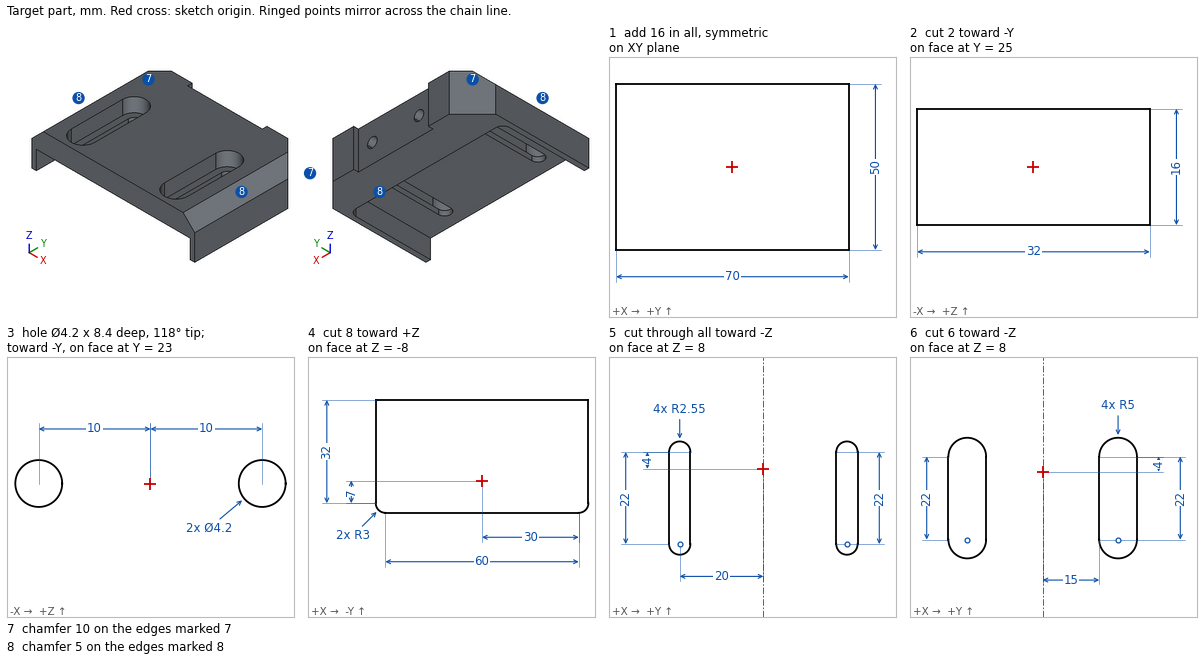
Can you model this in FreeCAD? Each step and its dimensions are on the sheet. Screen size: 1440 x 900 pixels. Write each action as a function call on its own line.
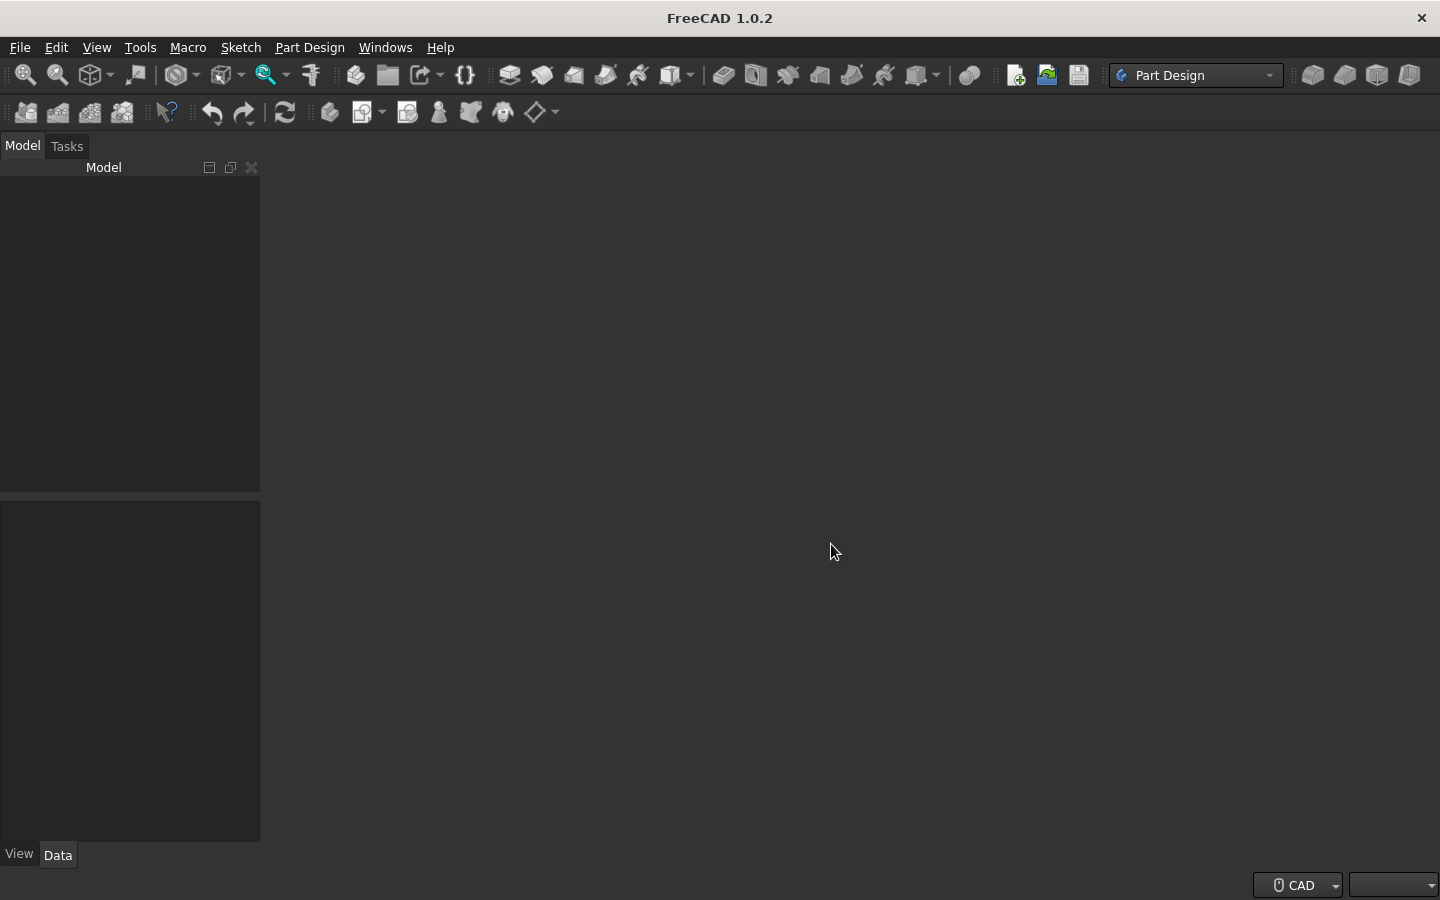
key(ctrl+n)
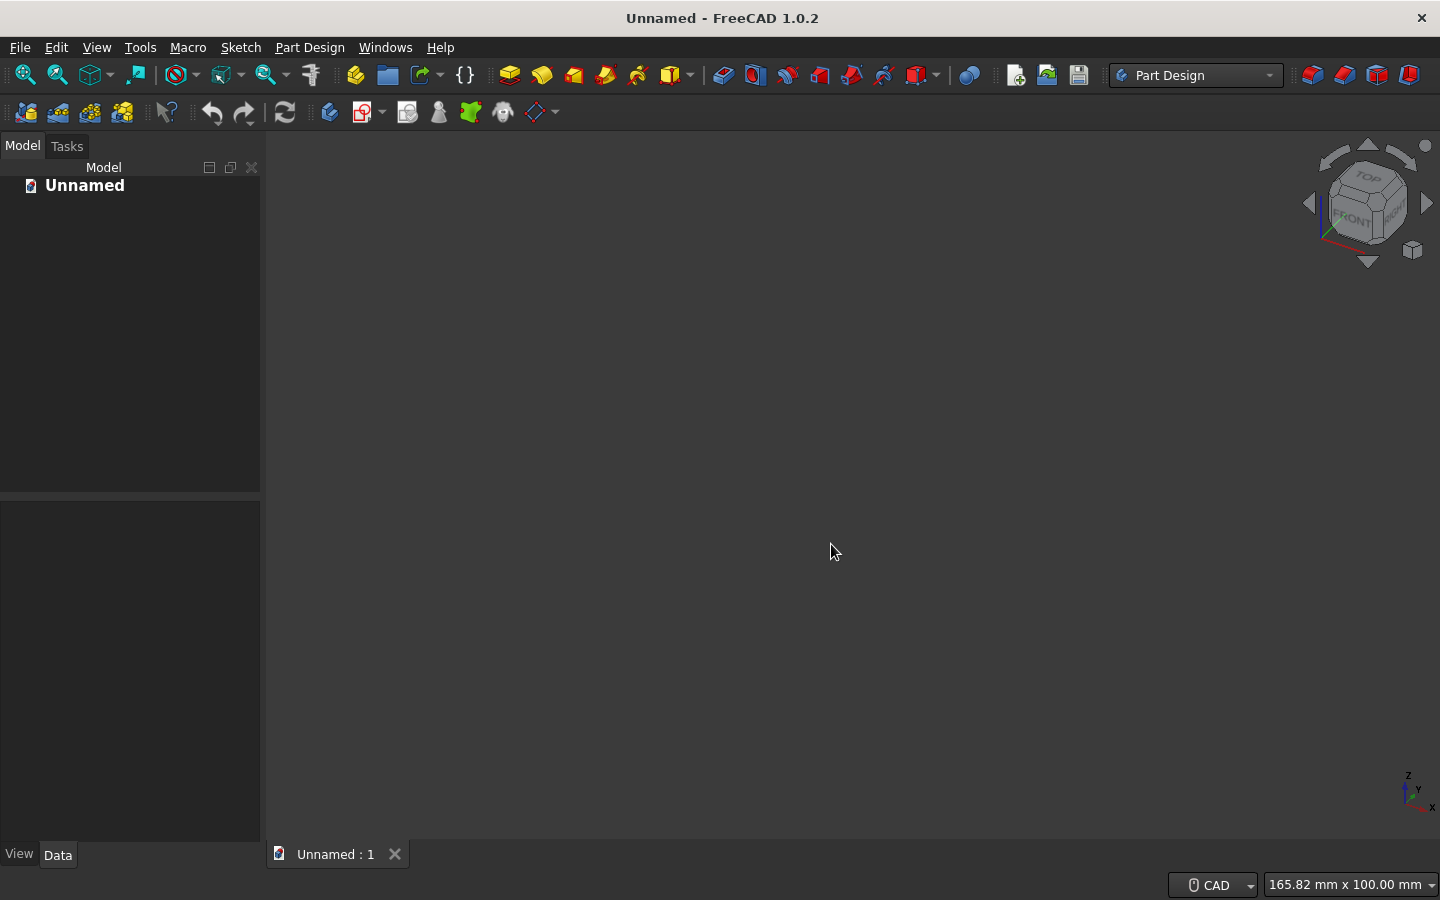
click(362, 112)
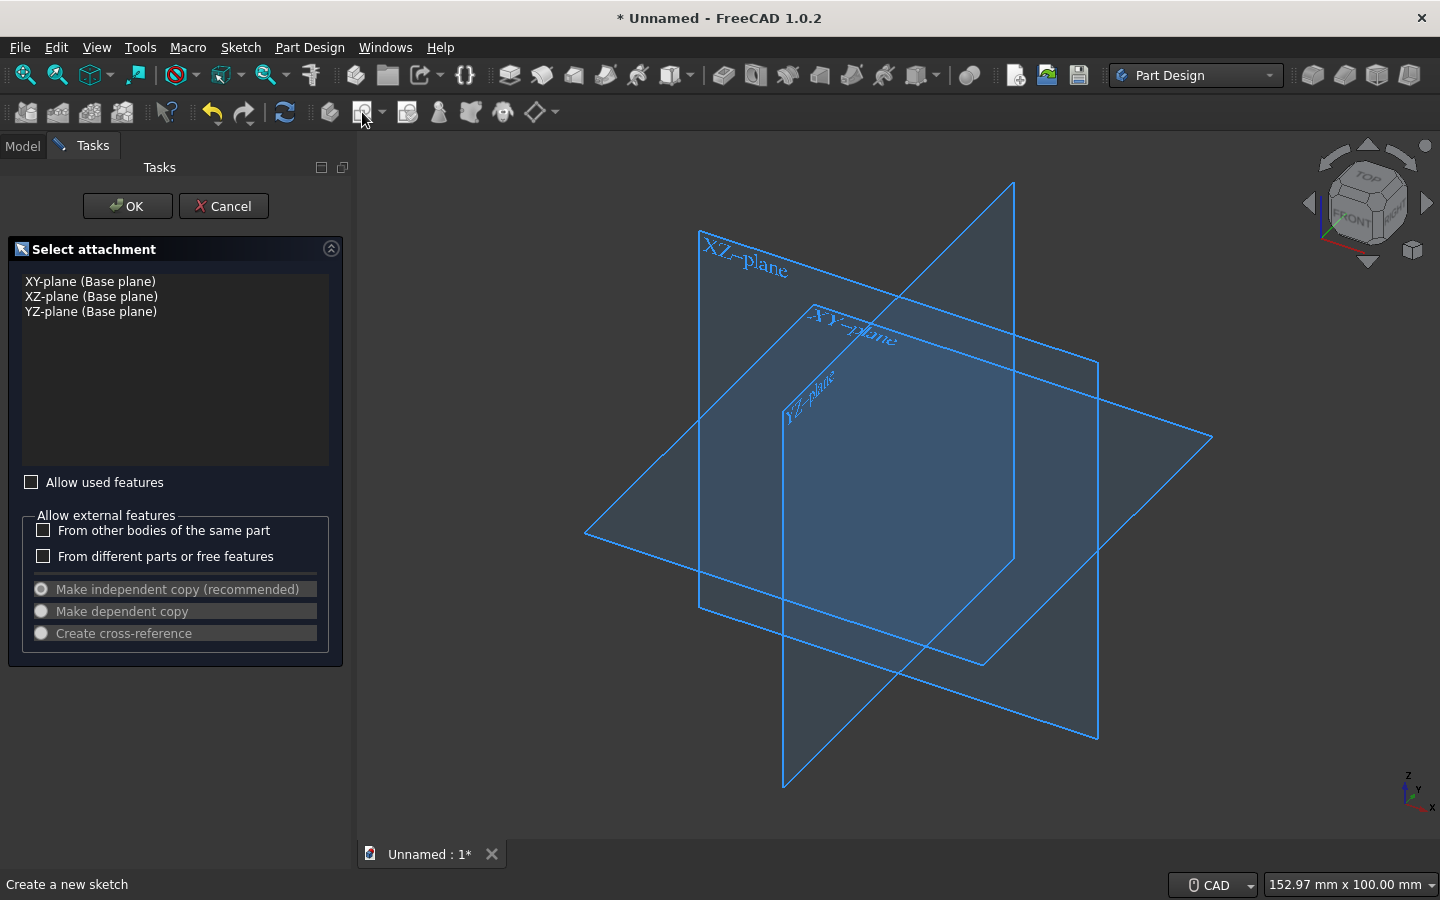
click(82, 282)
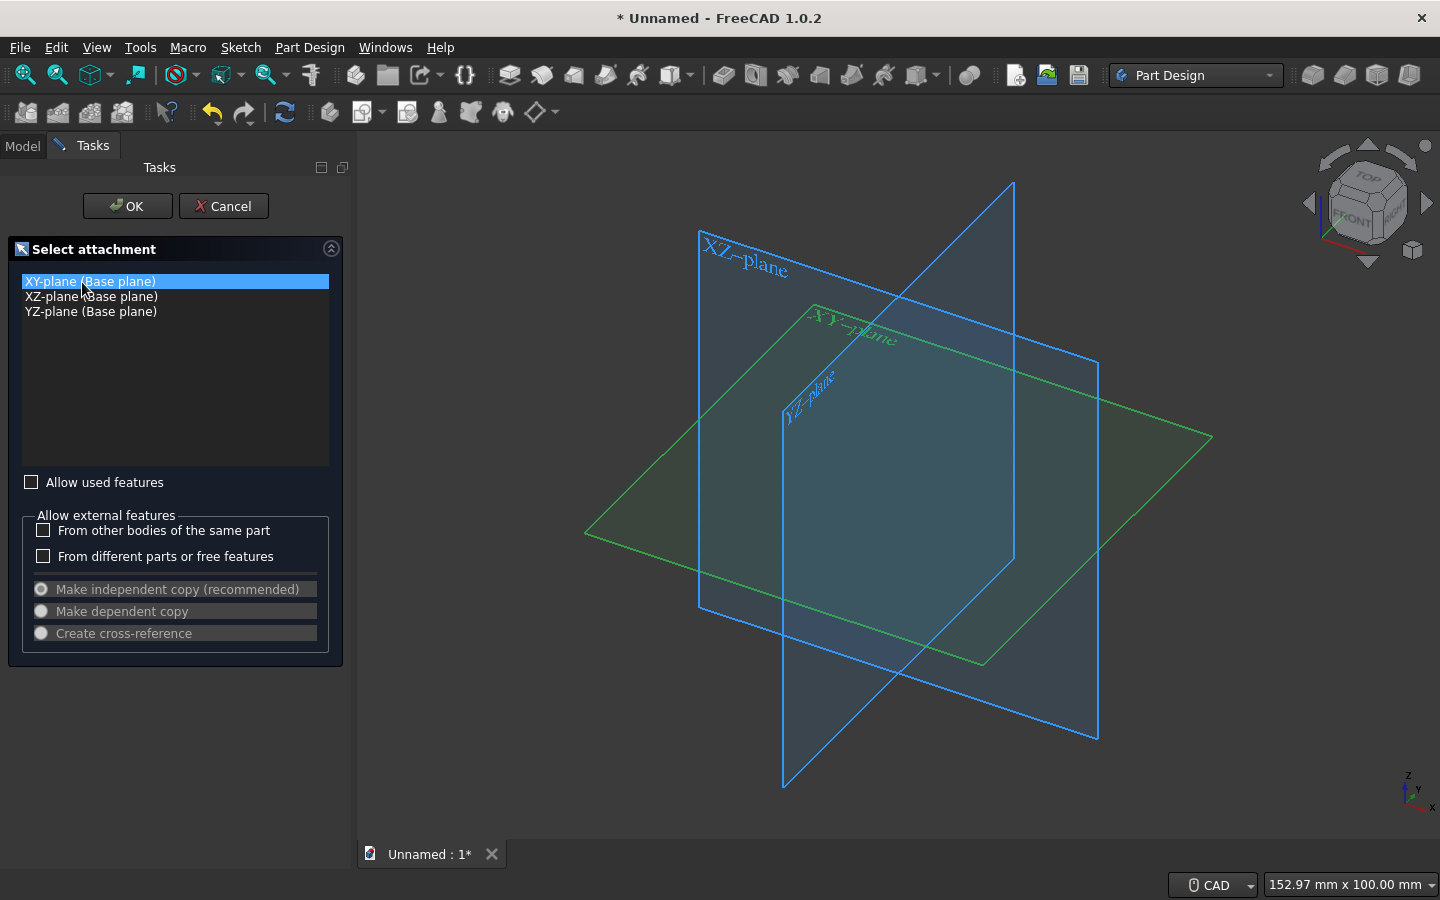
click(128, 206)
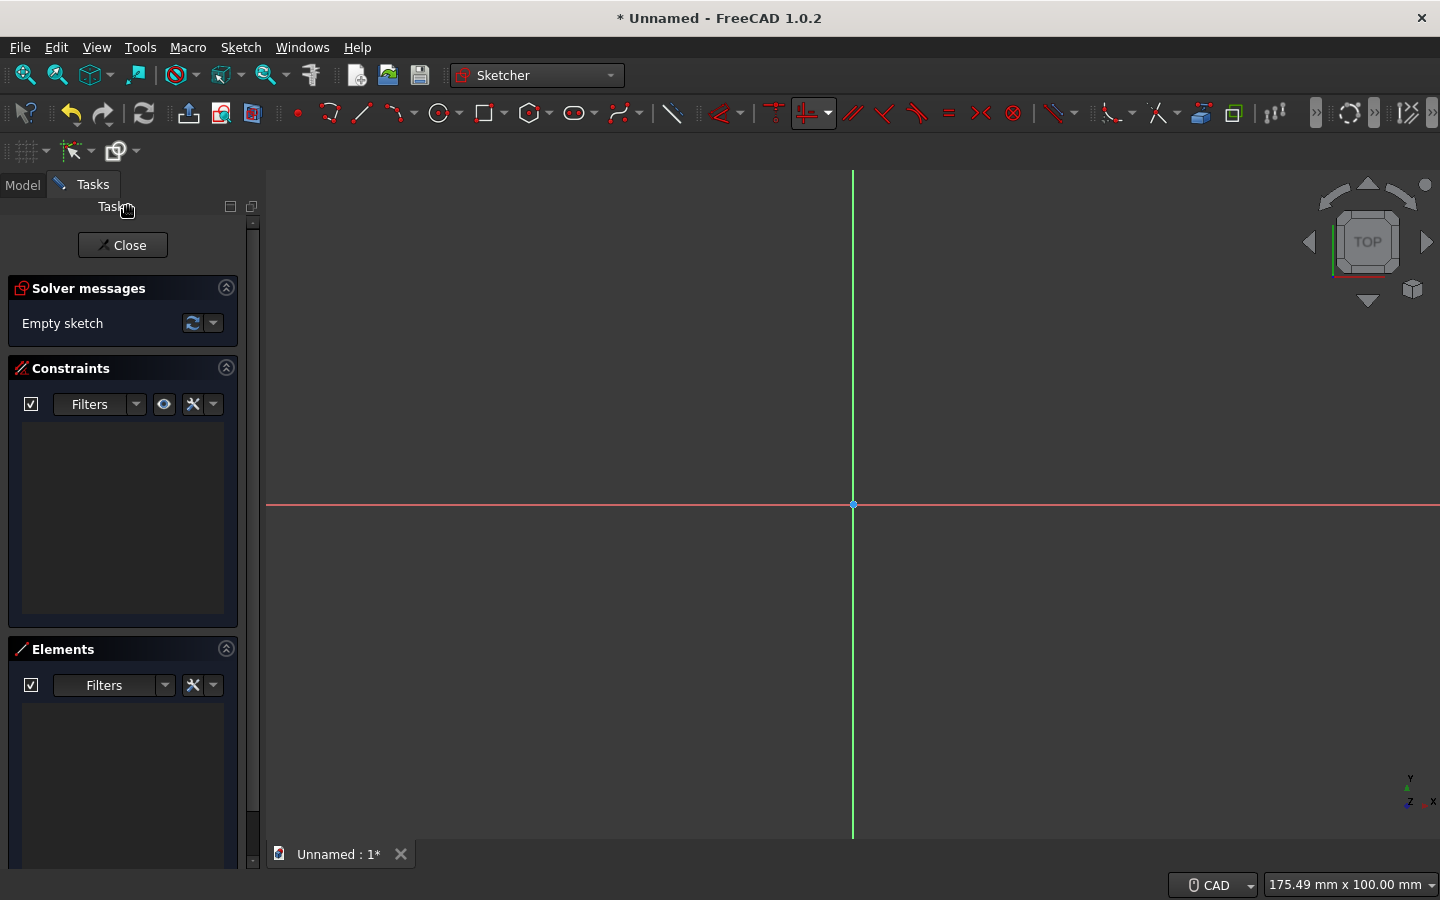
key(g)
key(v)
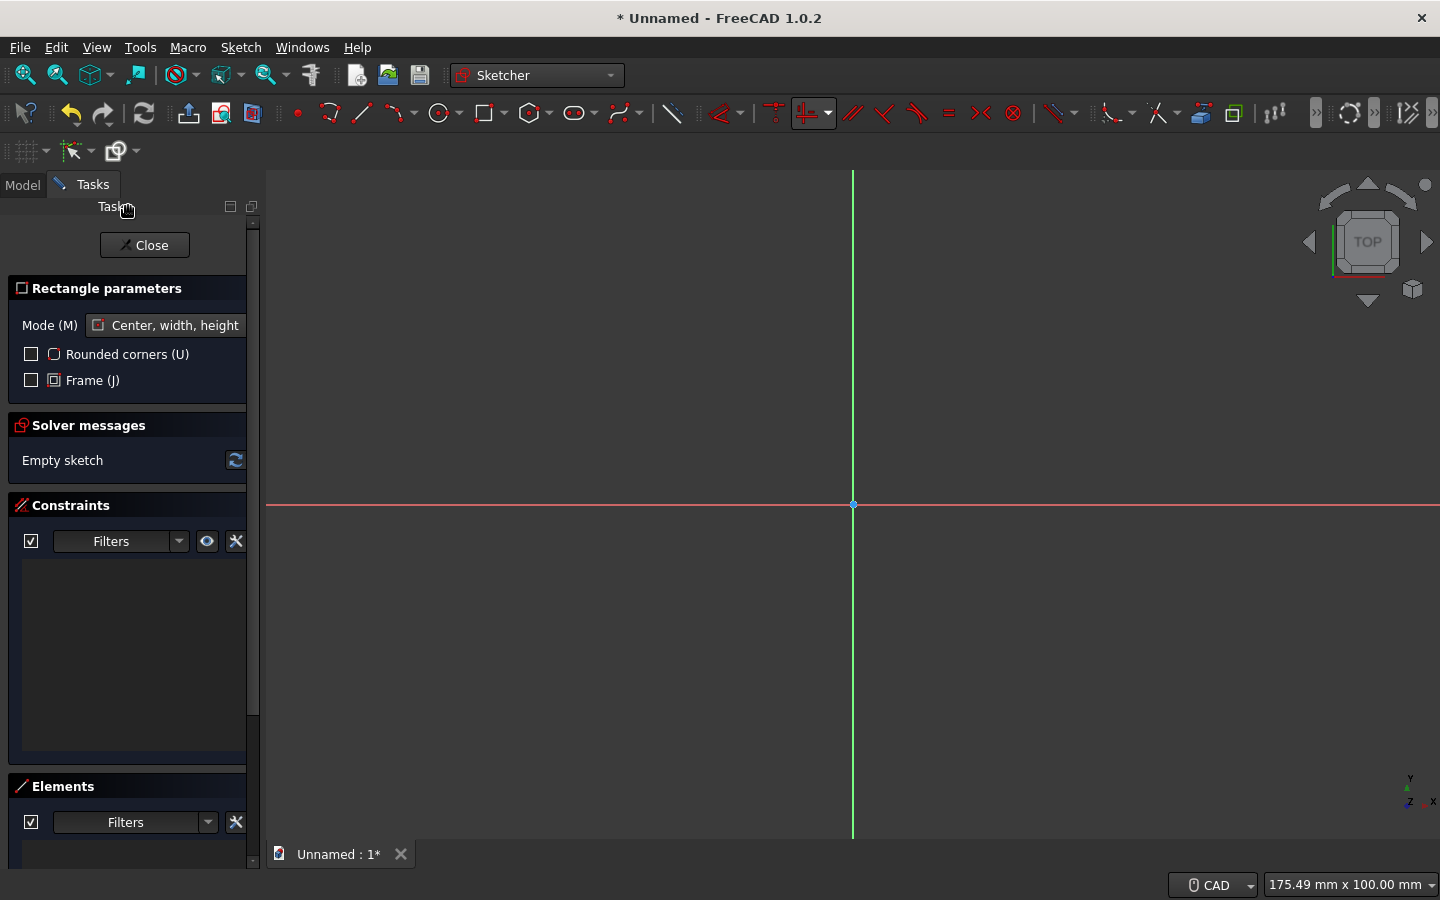
click(853, 504)
move(1087, 337)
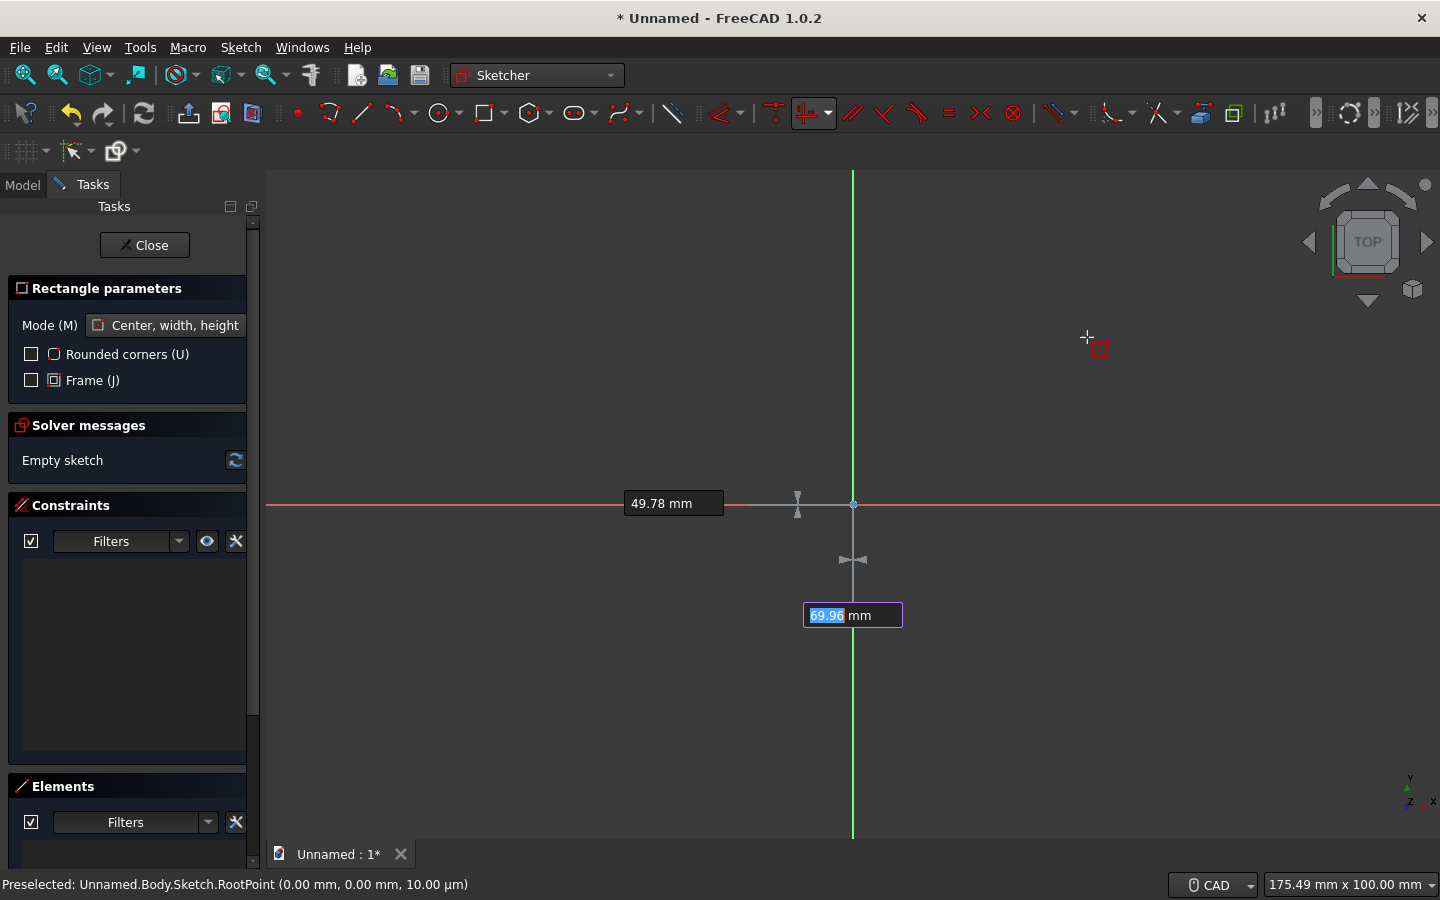
text(70)
key(Tab)
text(50)
key(Return)
key(Escape)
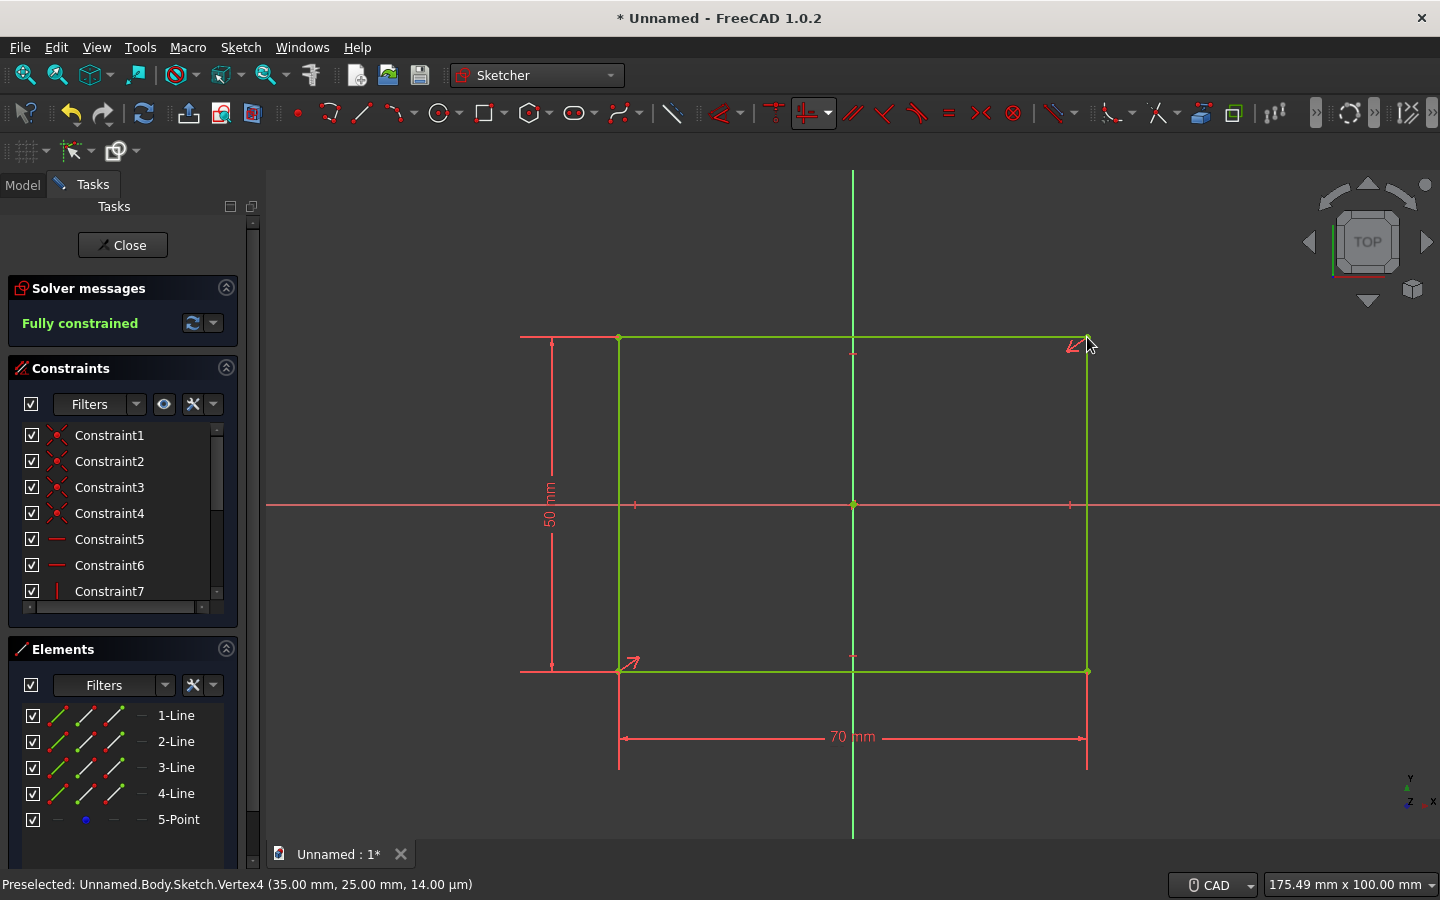
click(123, 245)